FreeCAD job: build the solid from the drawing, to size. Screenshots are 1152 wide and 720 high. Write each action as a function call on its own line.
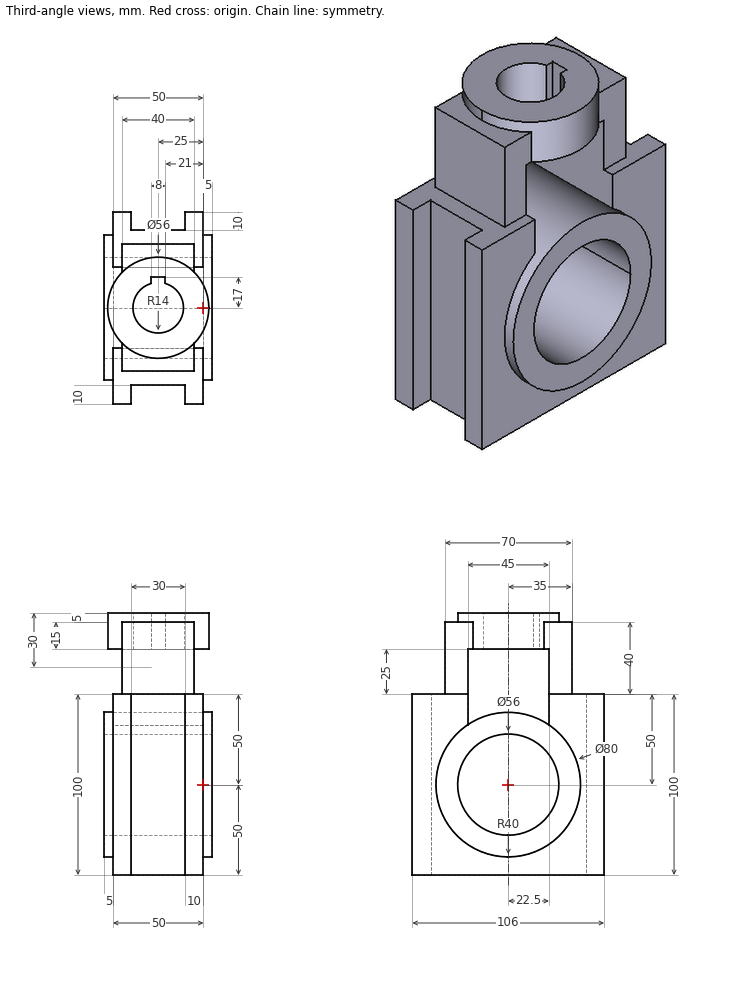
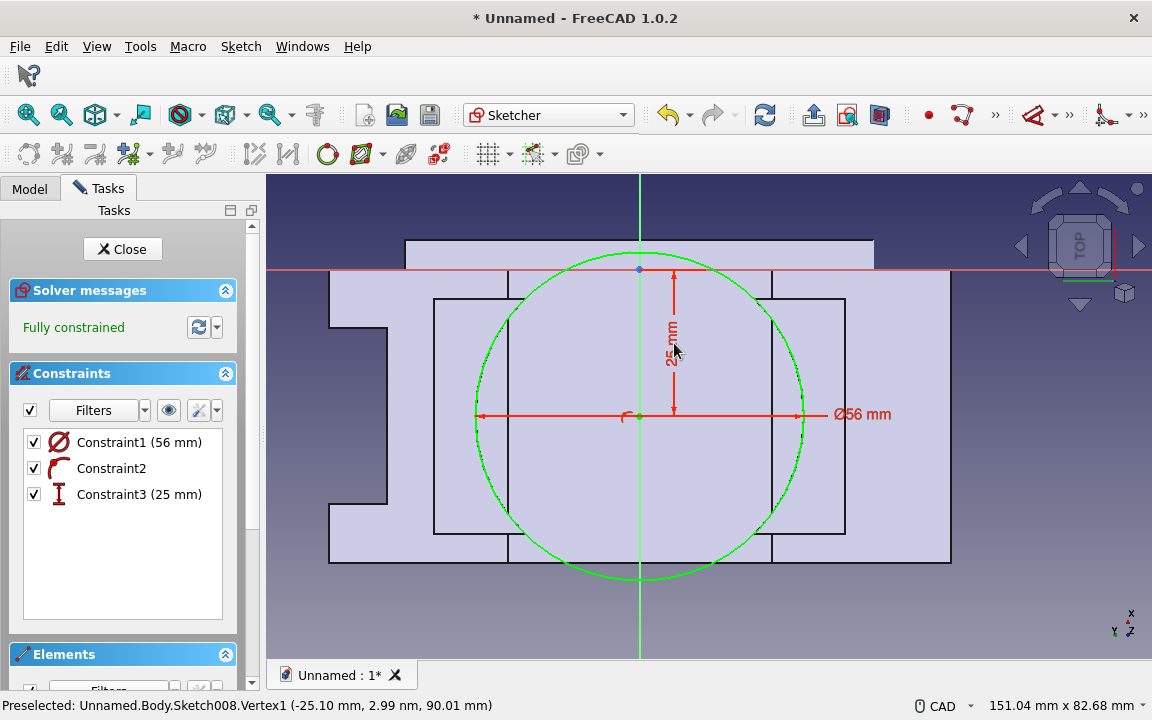
click(123, 249)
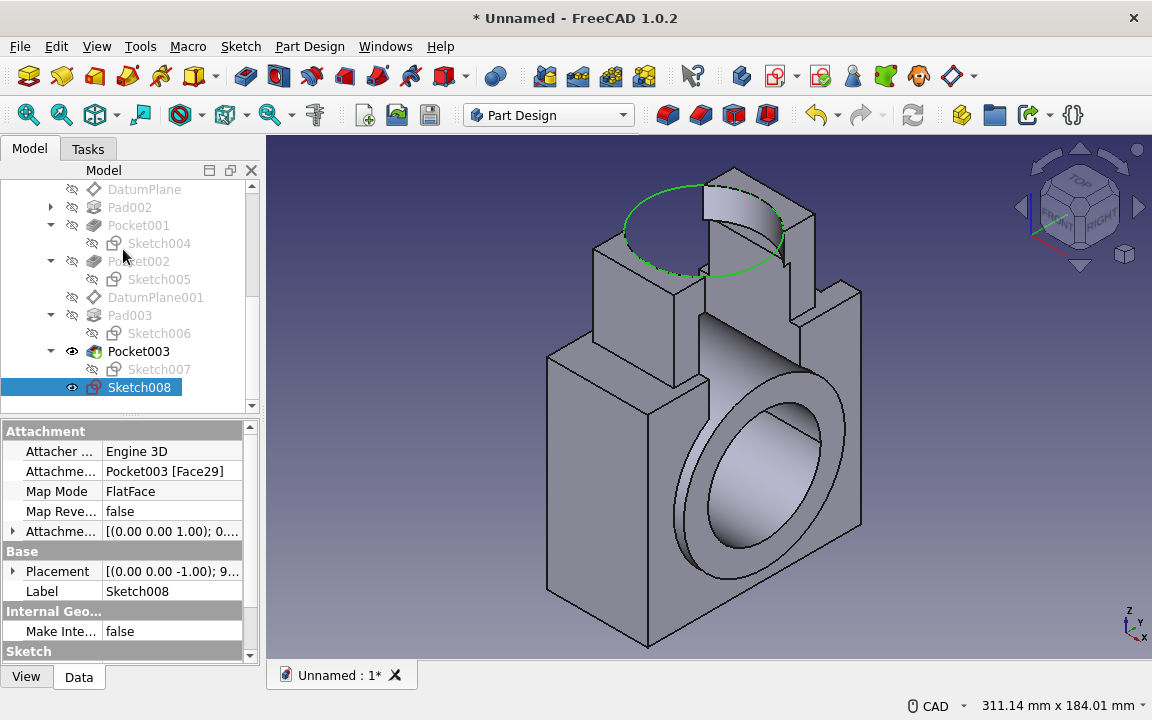
click(29, 76)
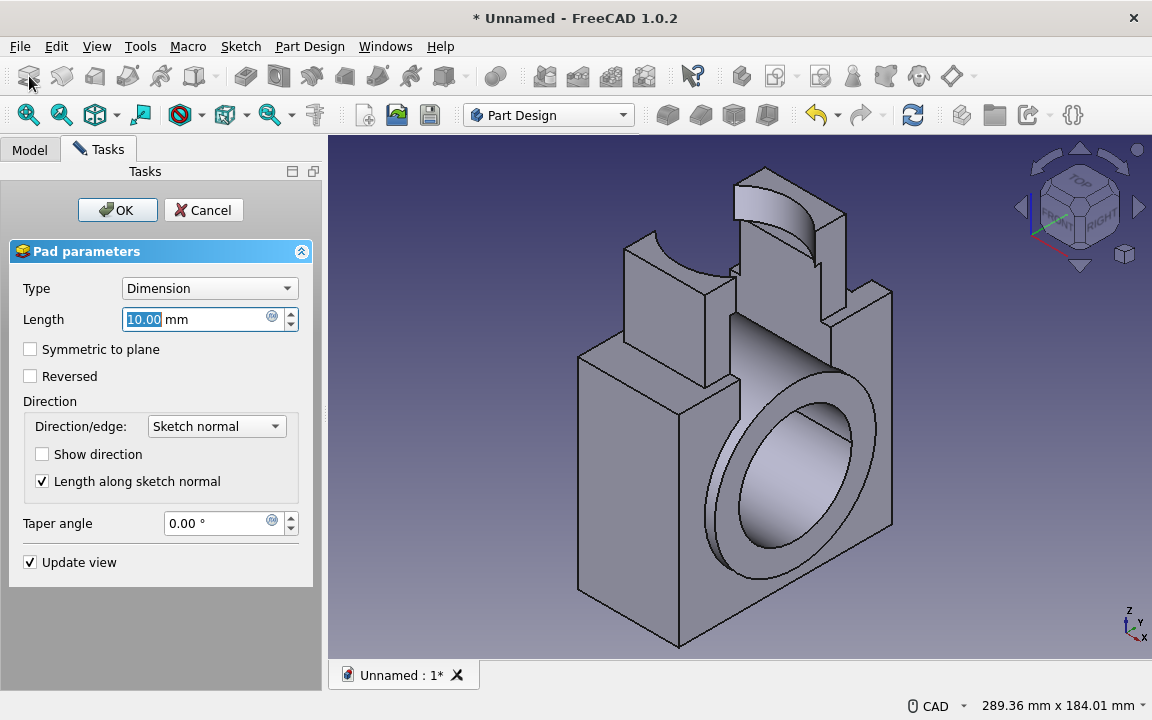
click(210, 288)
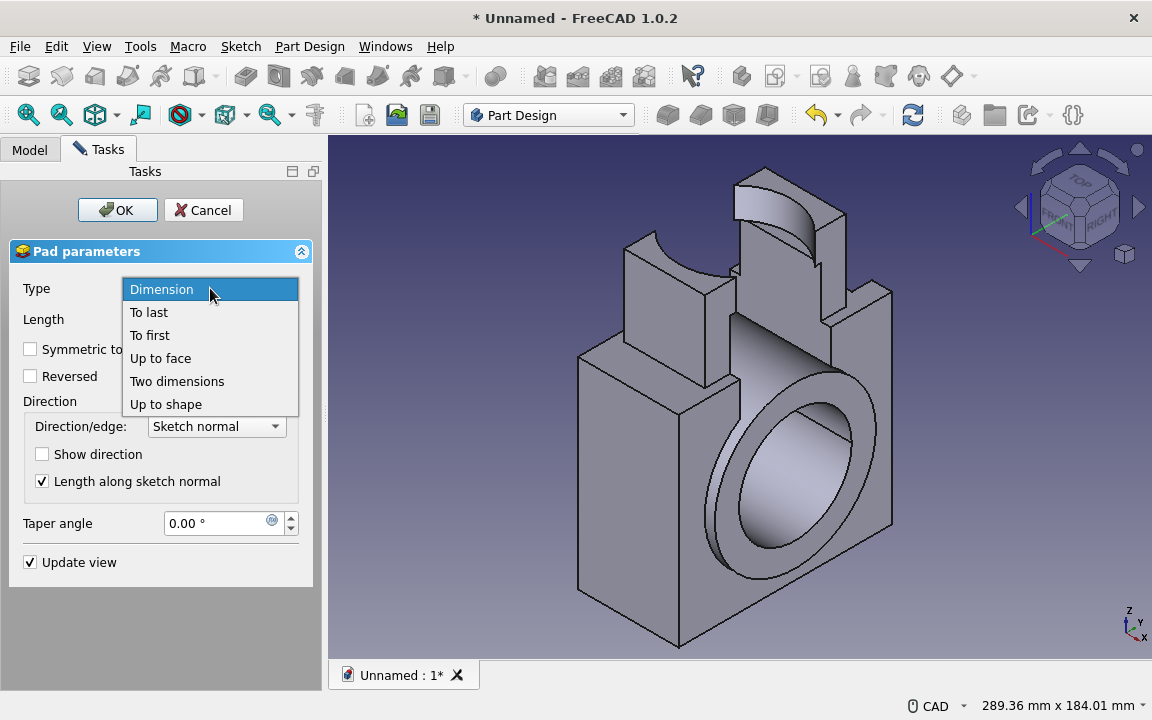
click(208, 382)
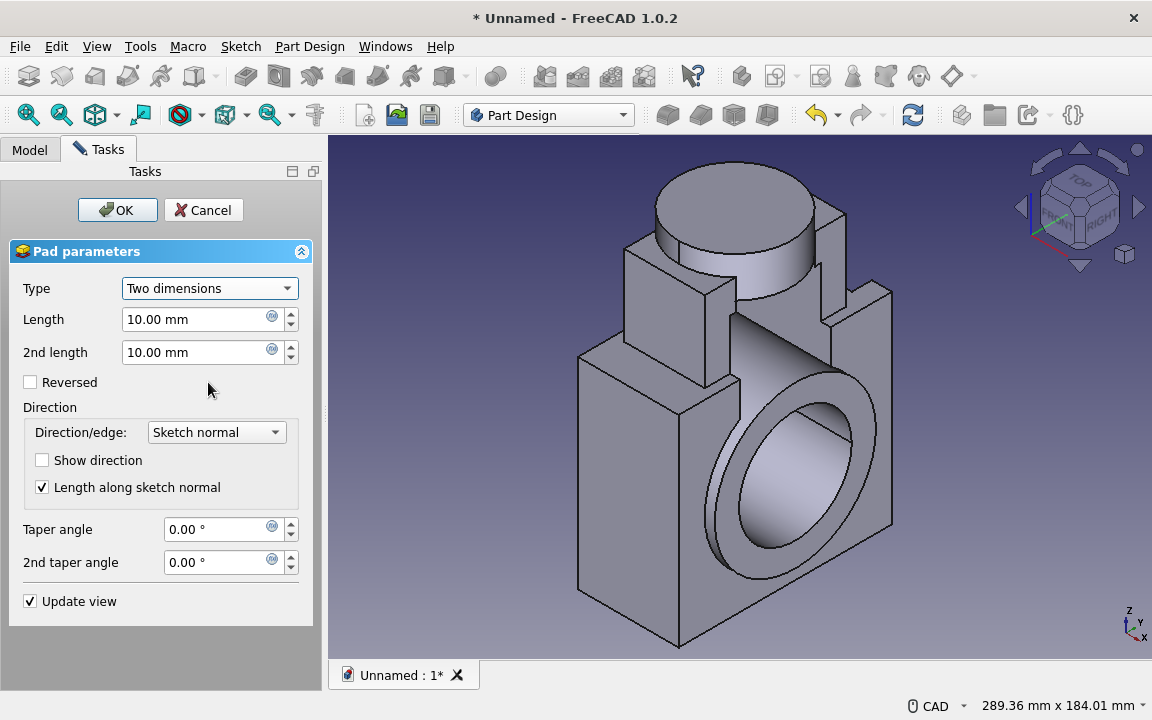
triple_click(204, 320)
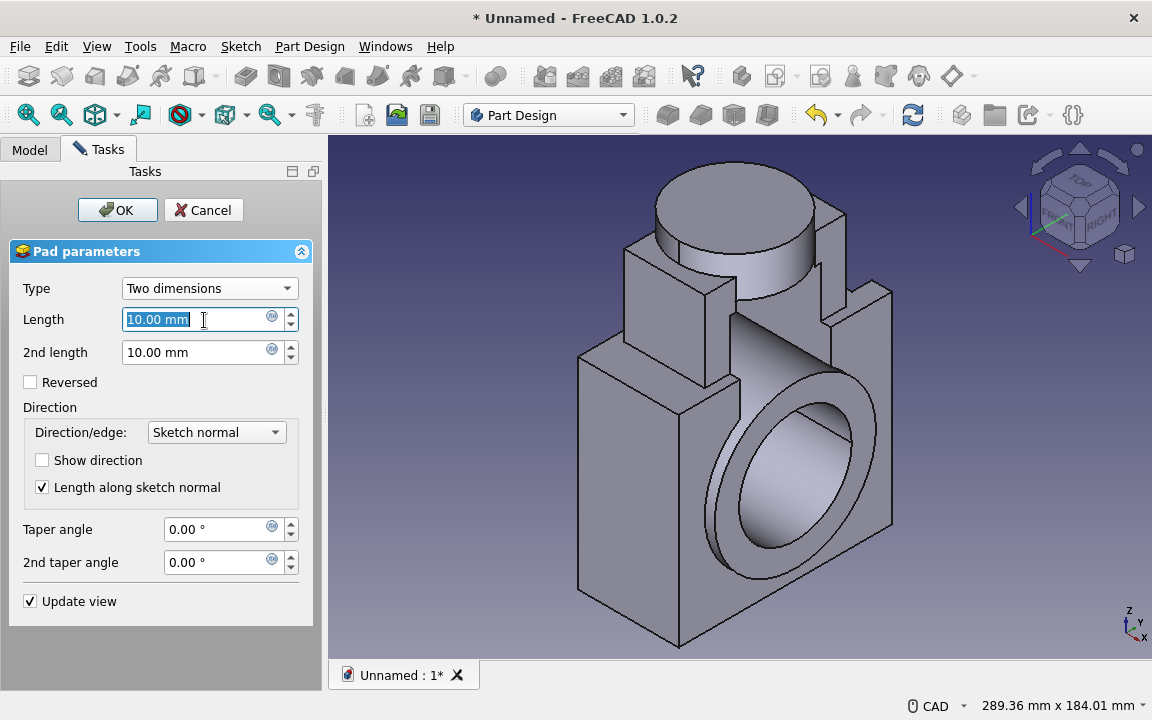
text(5)
key(Tab)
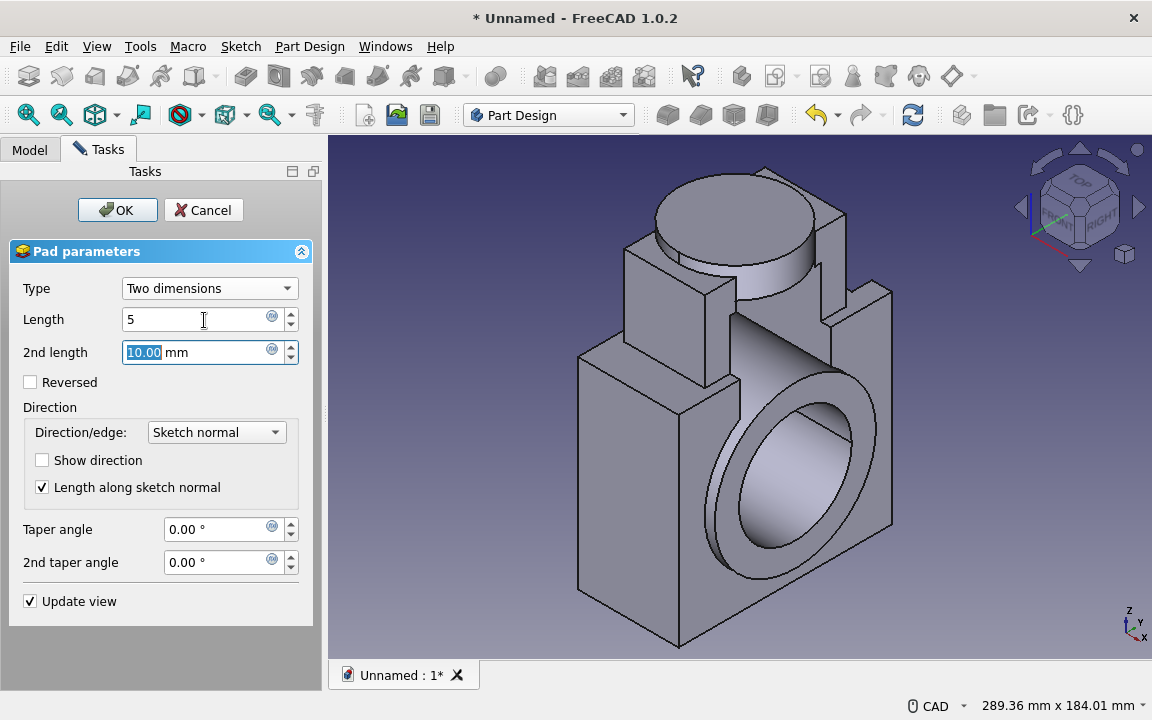
text(15)
key(Tab)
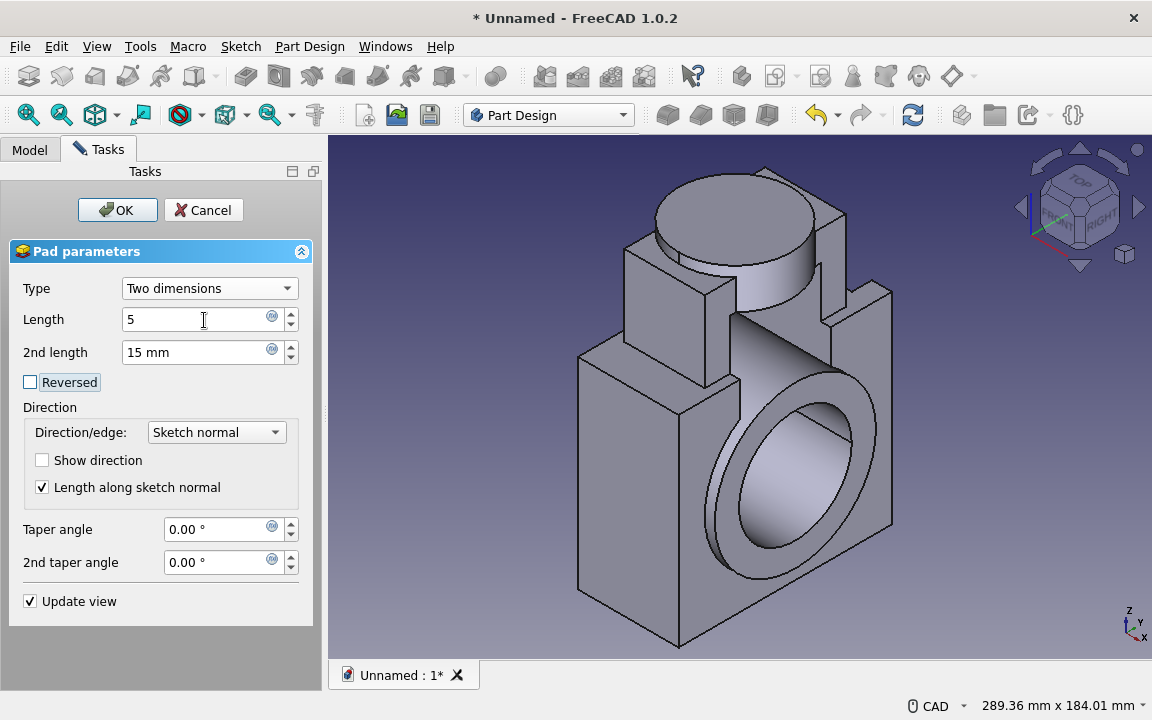
click(118, 210)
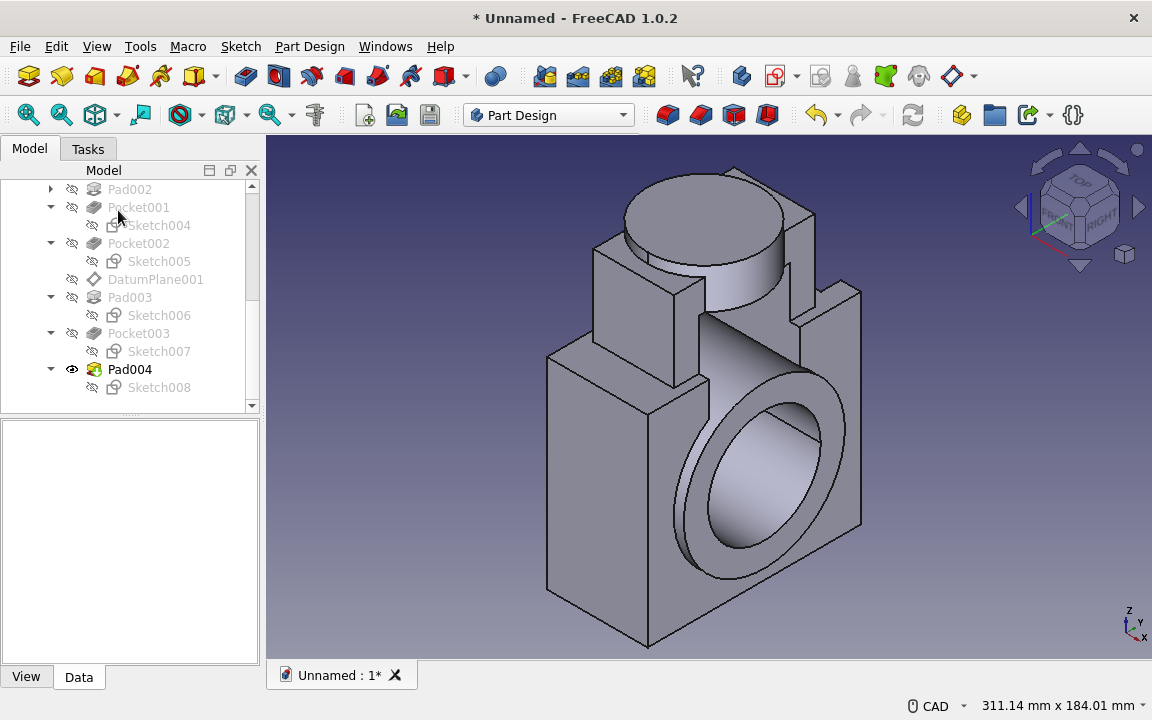
click(29, 116)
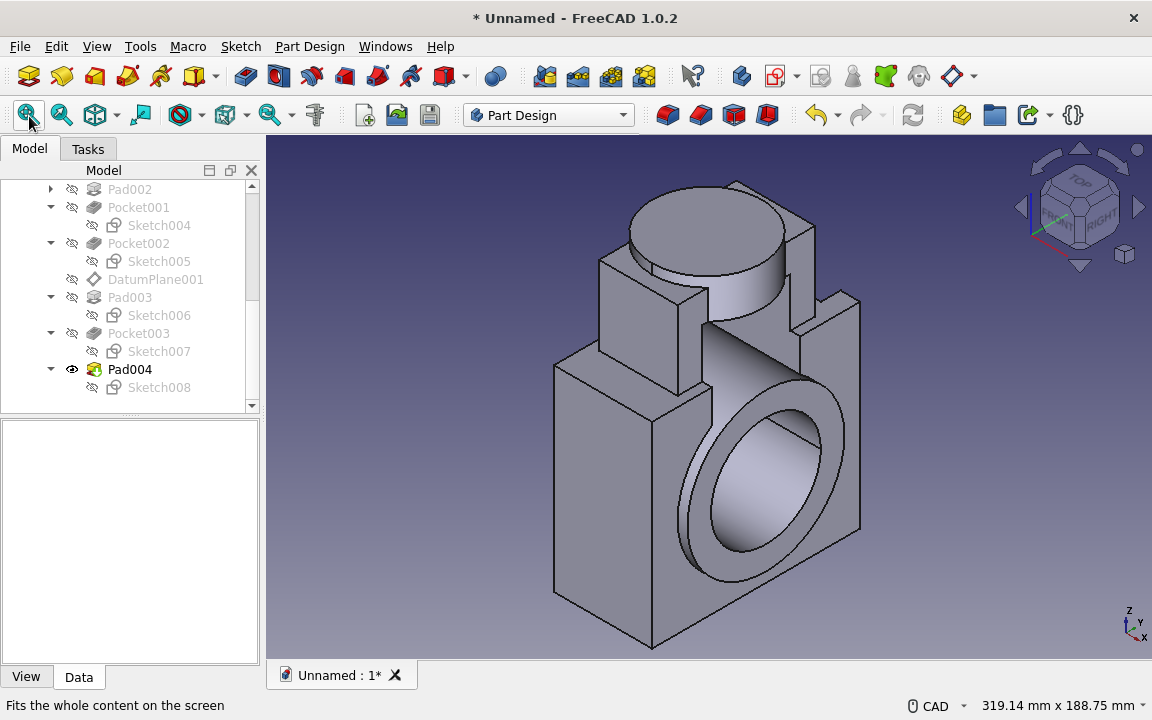
click(707, 231)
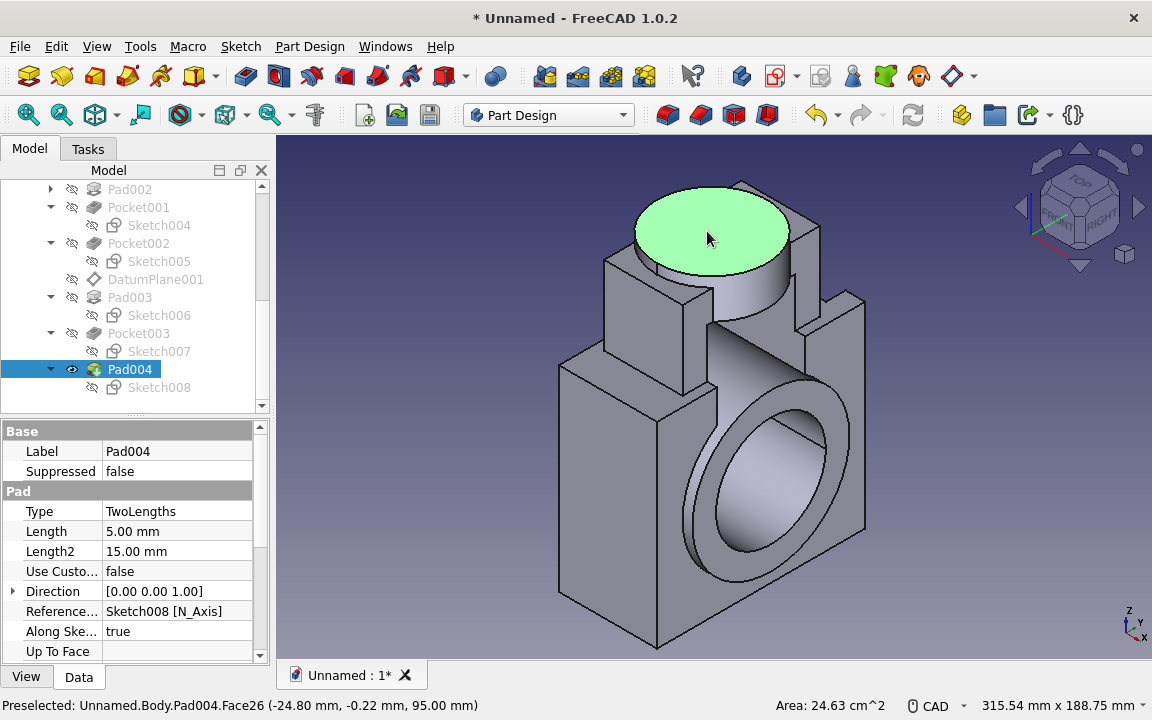
click(774, 76)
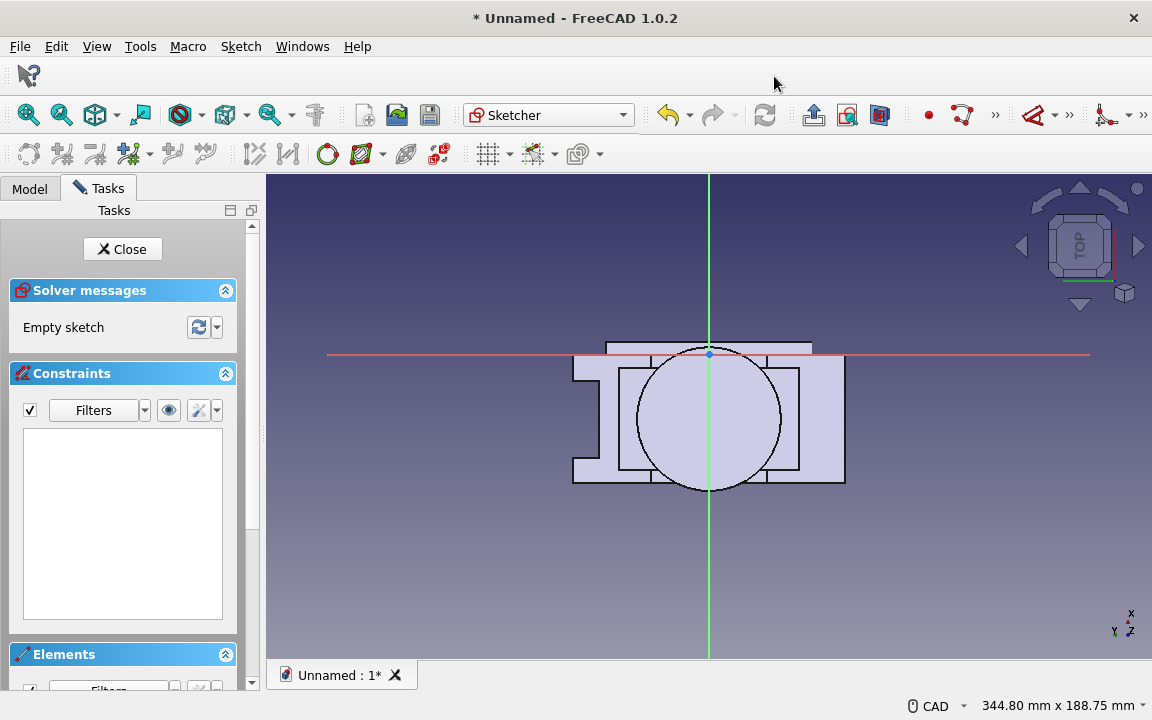
scroll(726, 384, up, 7)